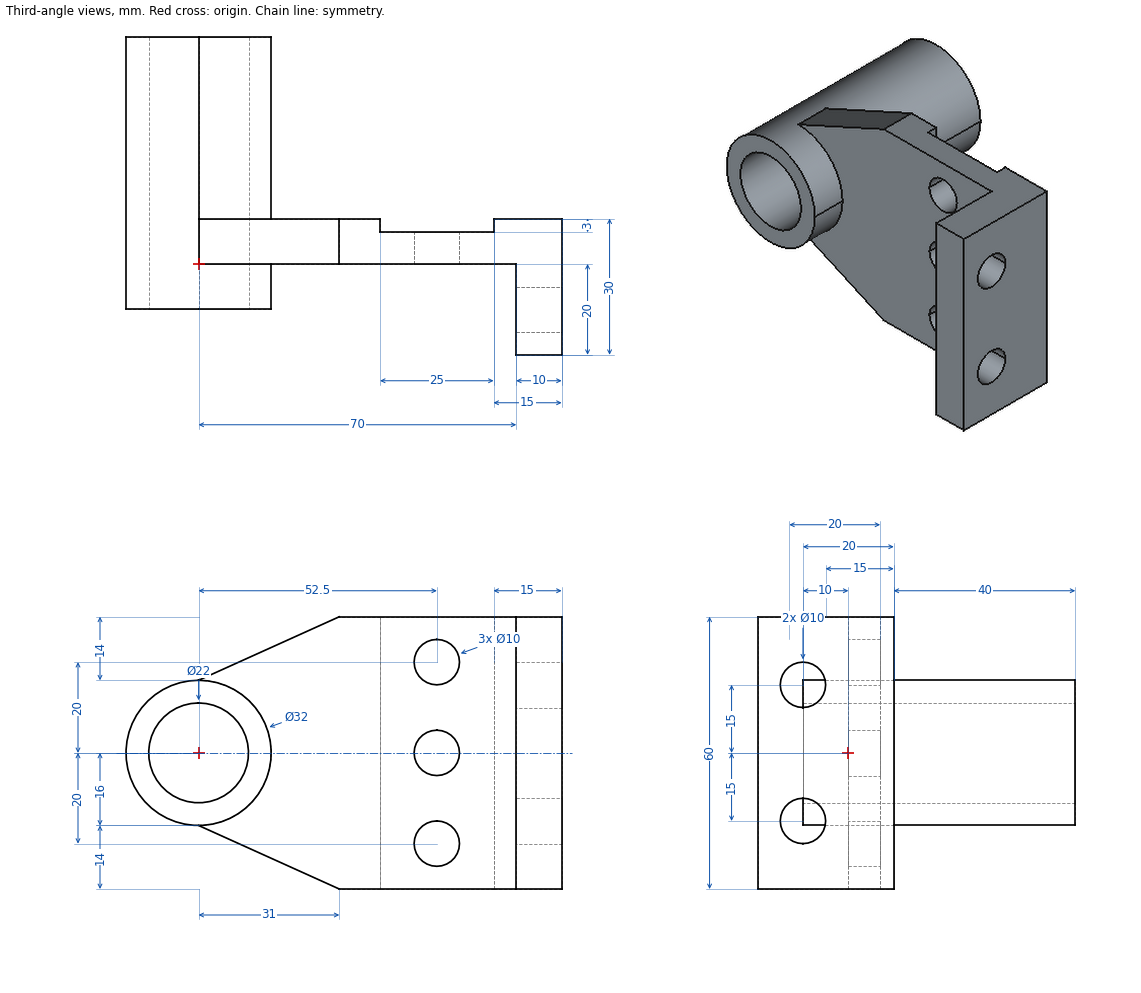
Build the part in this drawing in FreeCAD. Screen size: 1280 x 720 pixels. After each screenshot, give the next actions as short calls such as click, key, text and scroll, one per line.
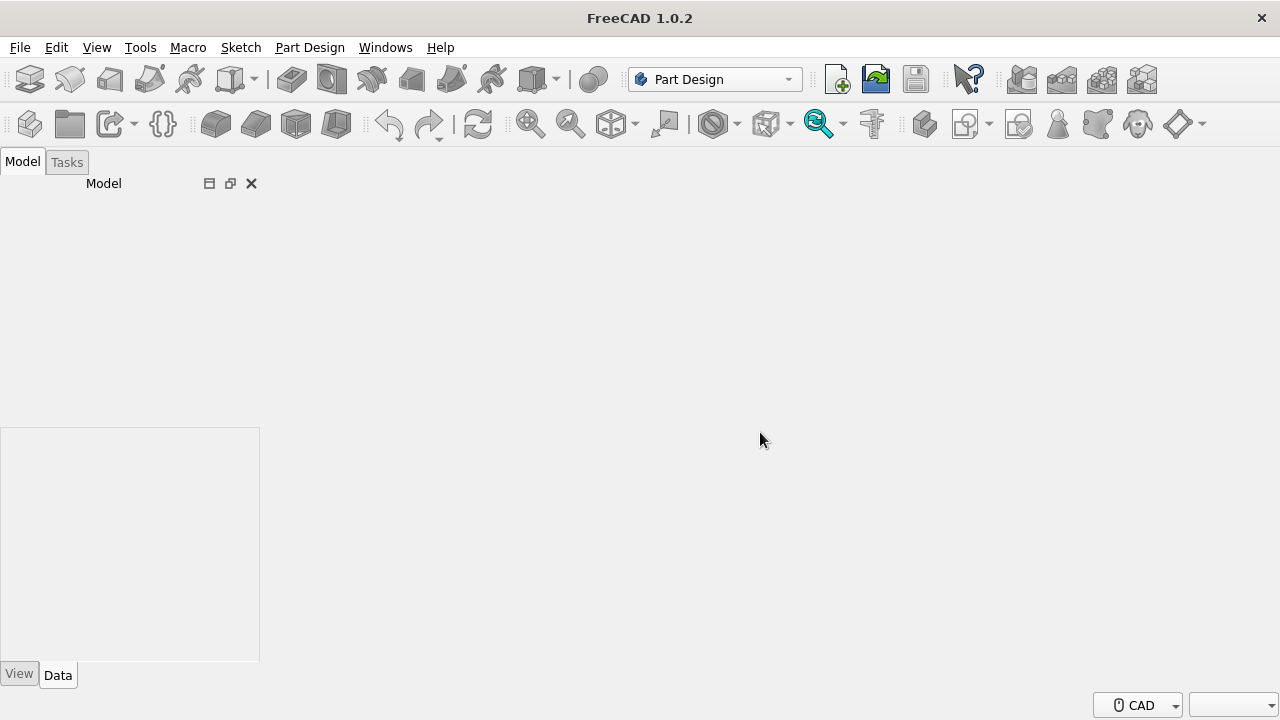
click(836, 80)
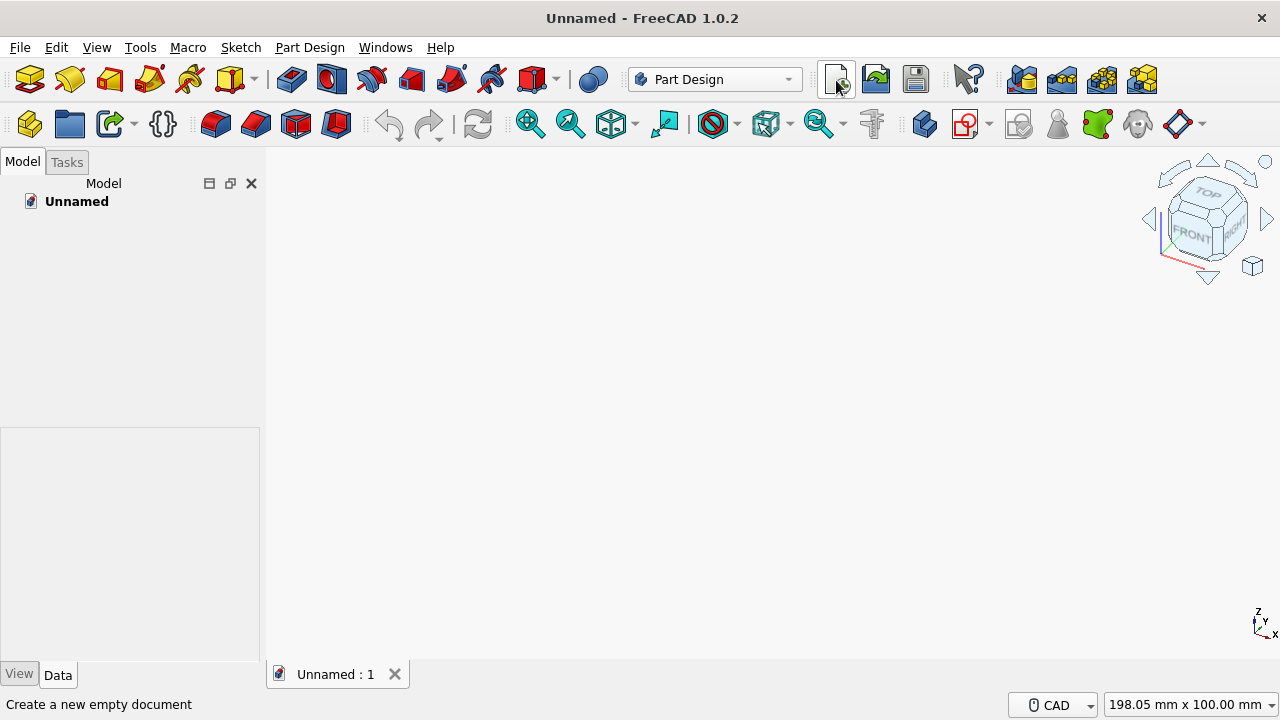
click(966, 124)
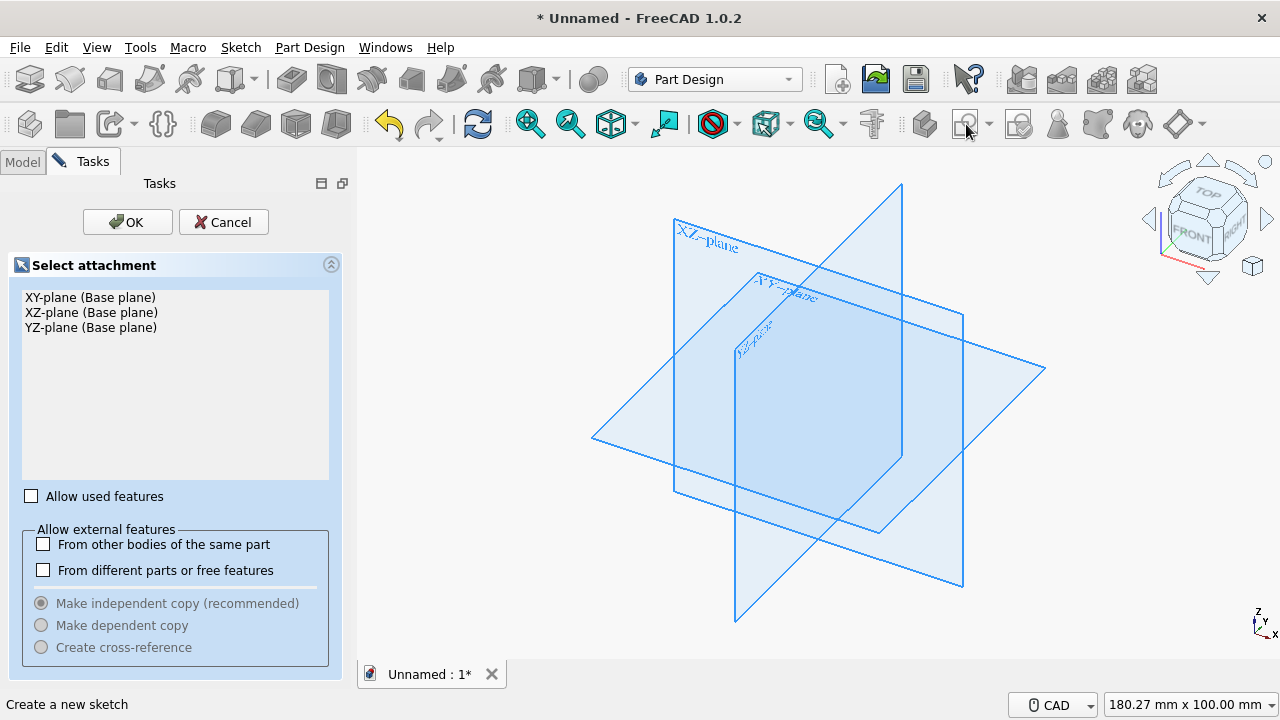
click(82, 298)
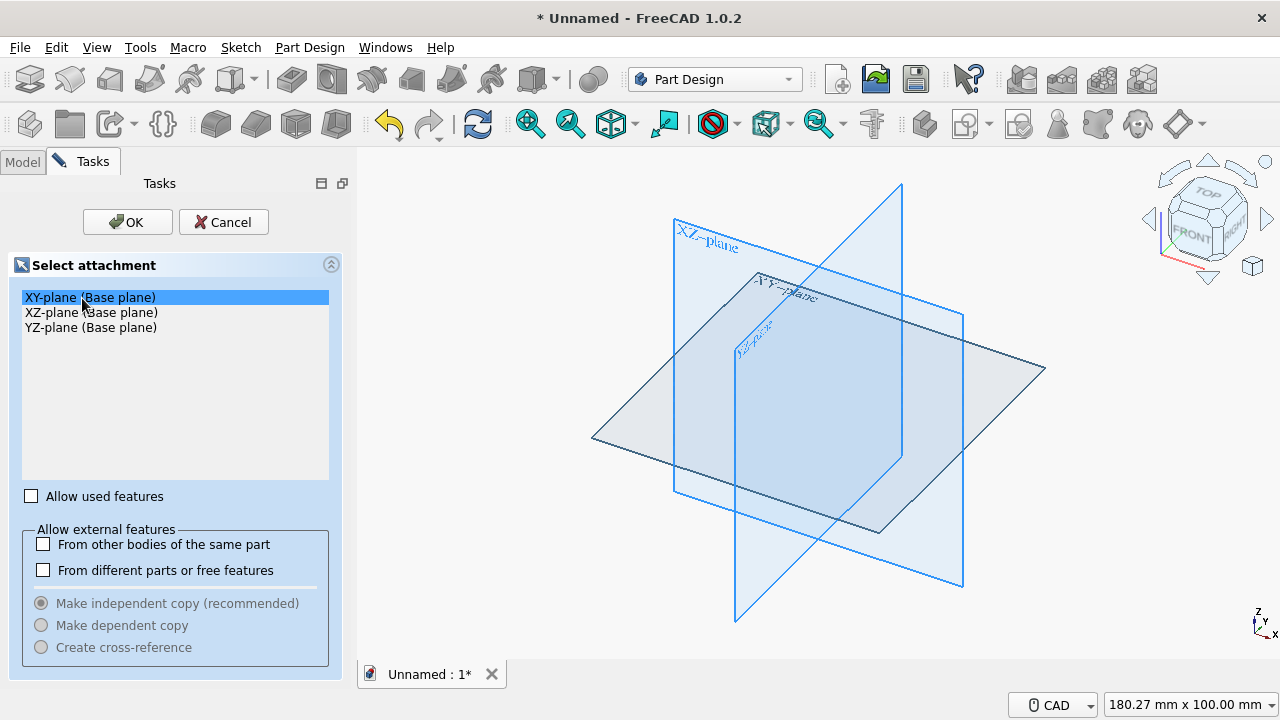
click(128, 222)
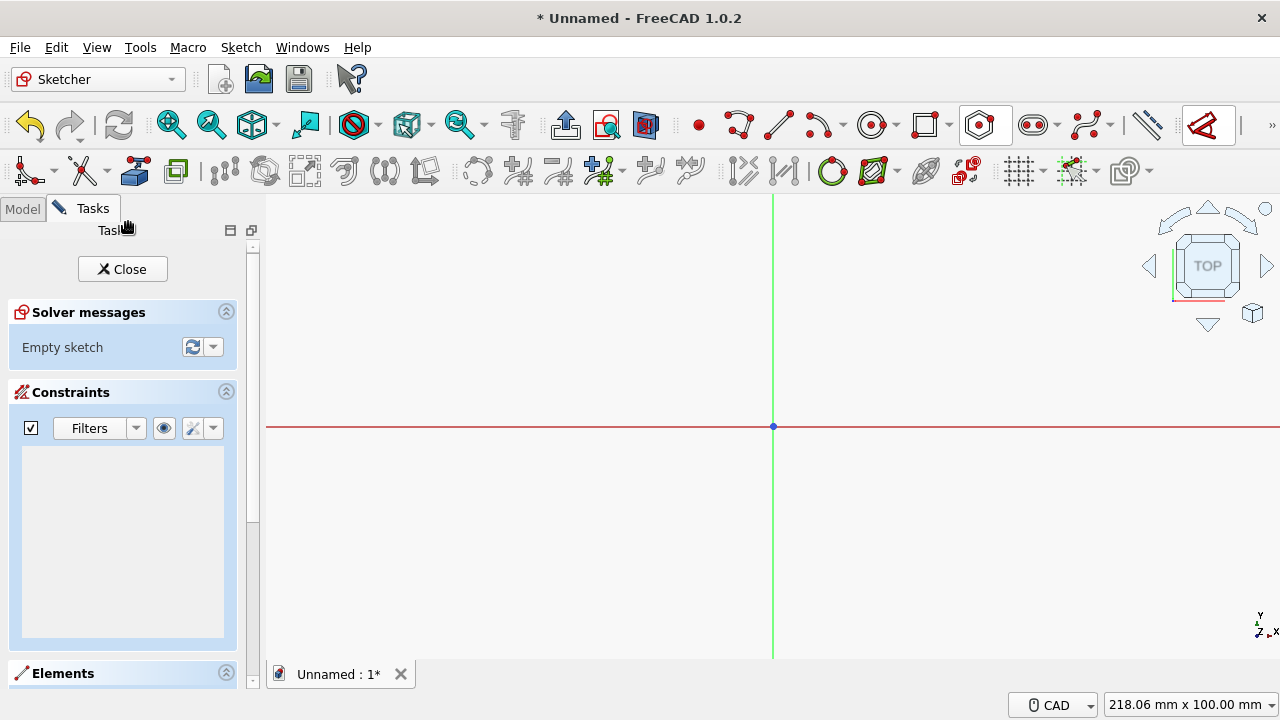
scroll(294, 321, down, 1)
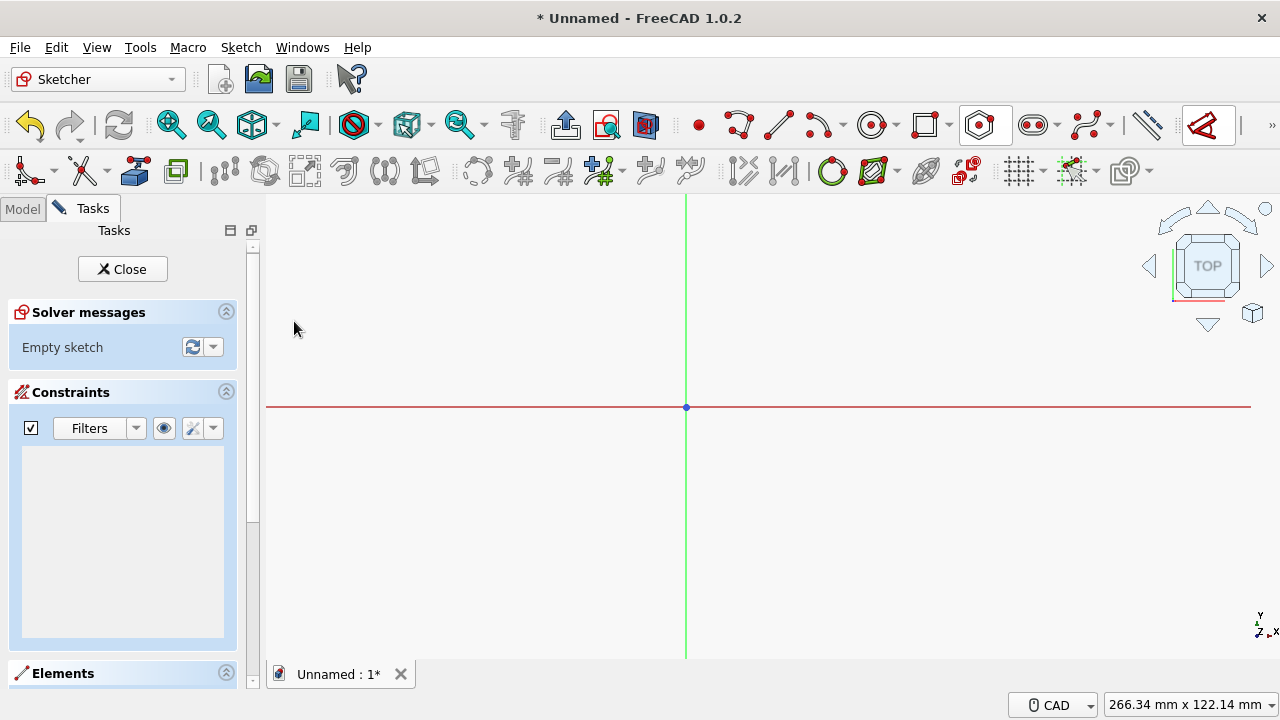
scroll(1001, 426, up, 3)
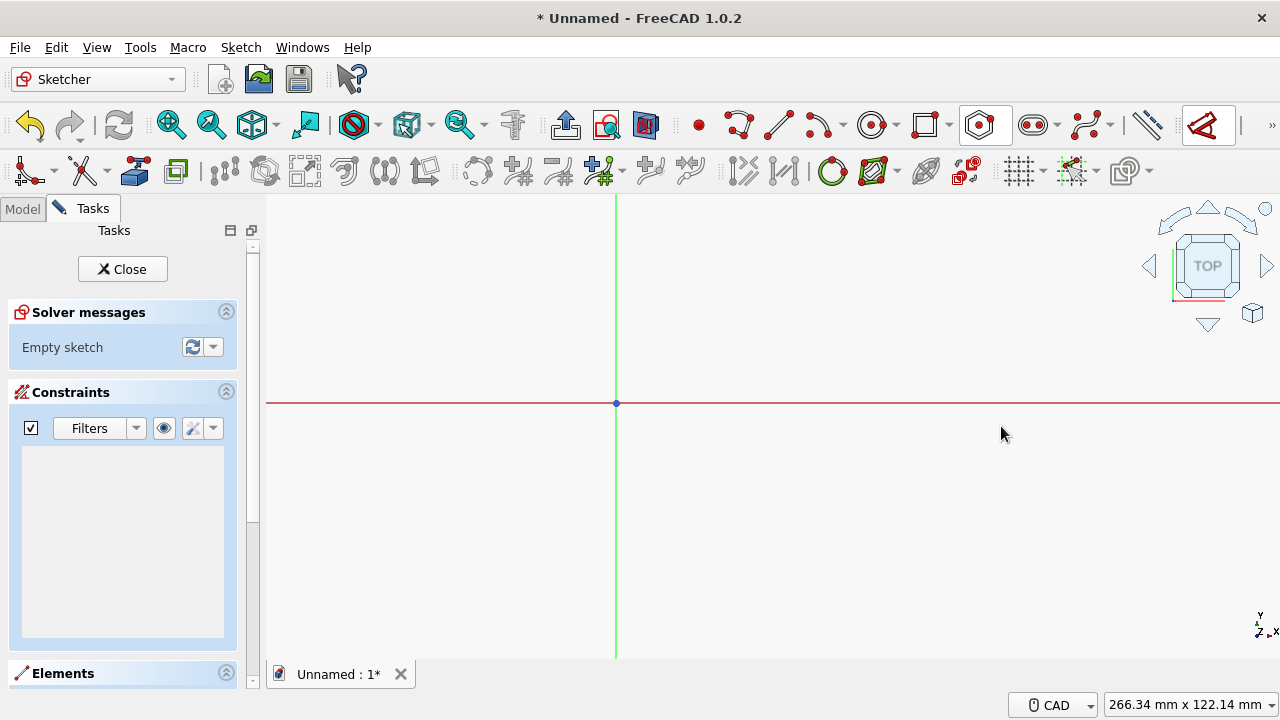
click(740, 126)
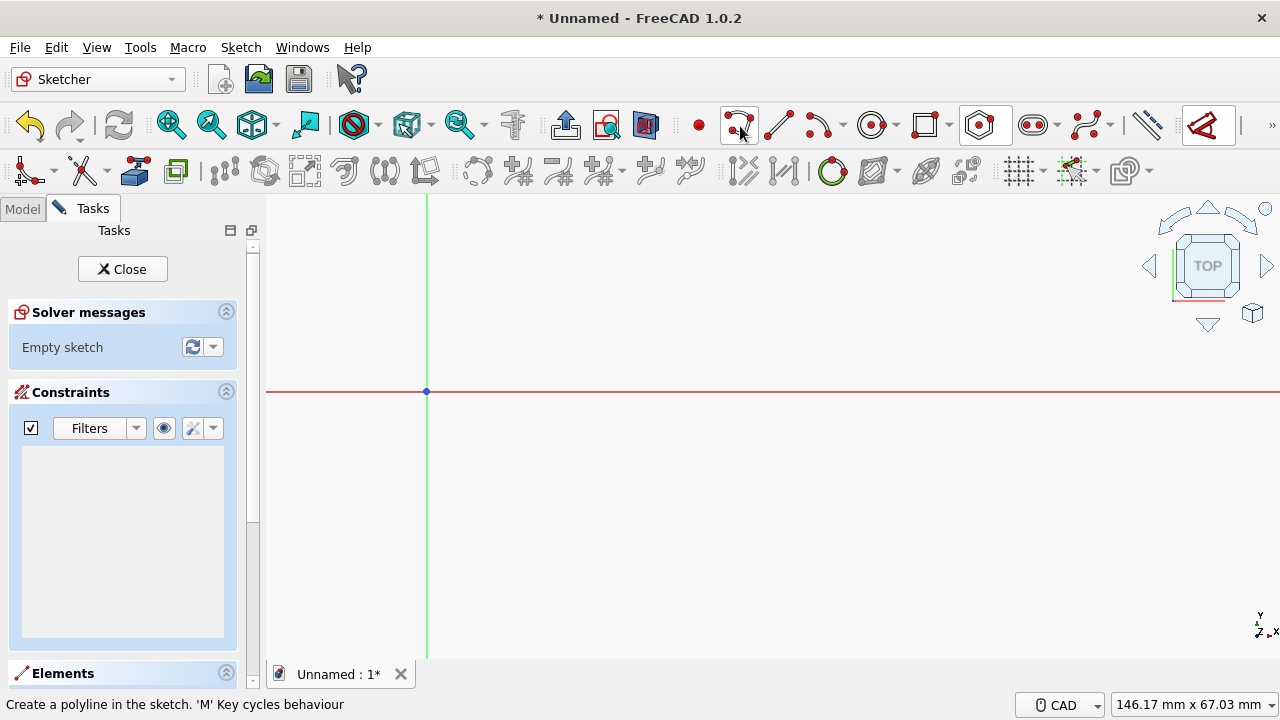
click(427, 392)
click(912, 401)
click(912, 530)
click(982, 530)
click(982, 322)
click(878, 322)
click(878, 343)
click(704, 343)
click(704, 322)
click(436, 322)
click(427, 392)
key(Escape)
key(Escape)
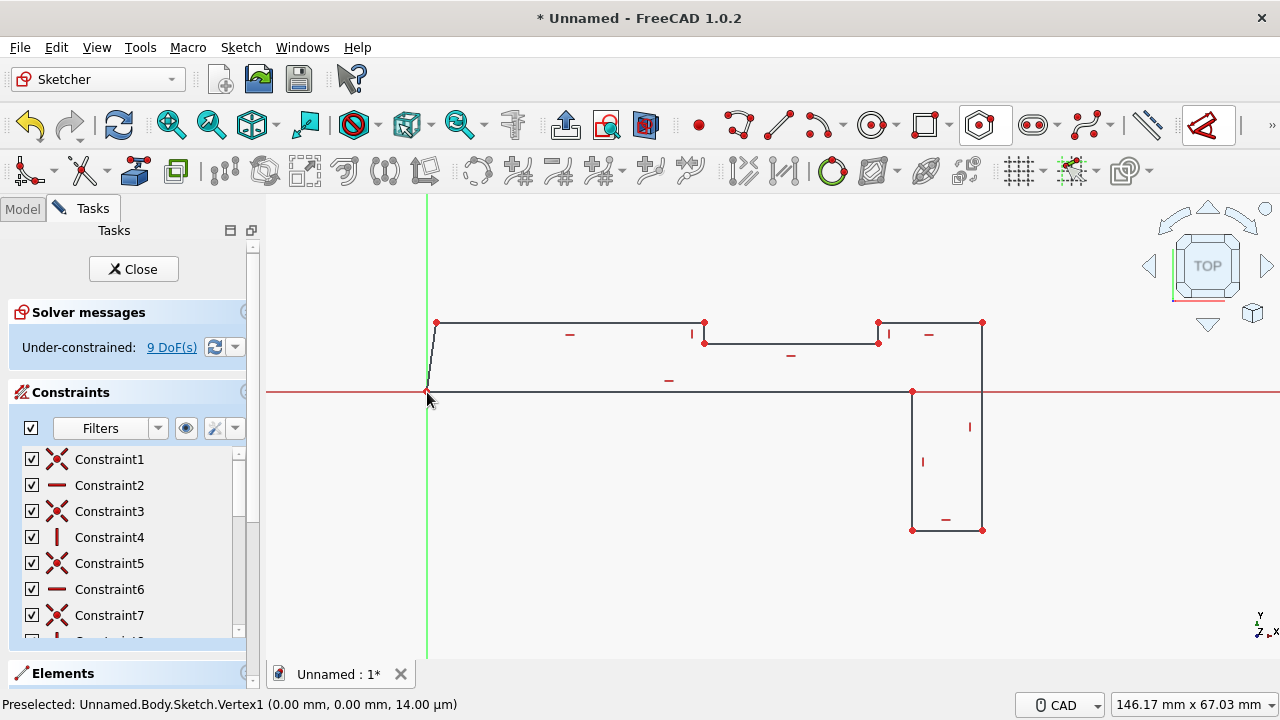
click(430, 371)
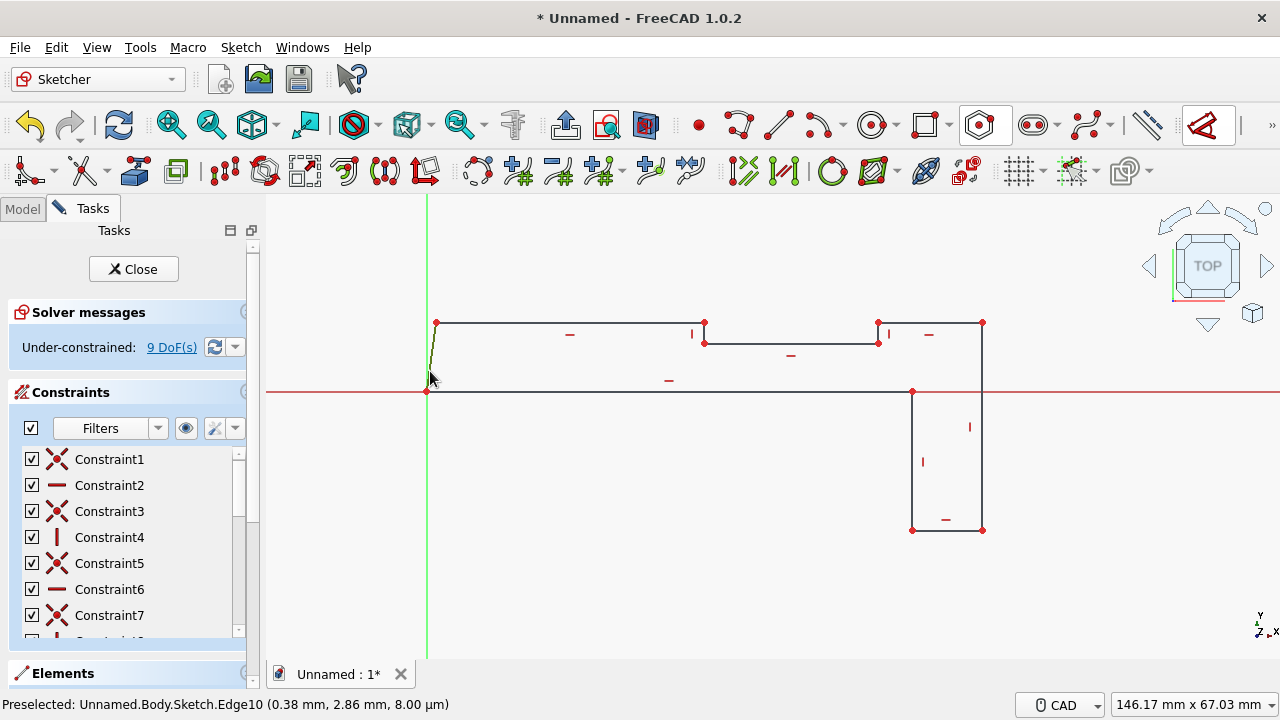
key(v)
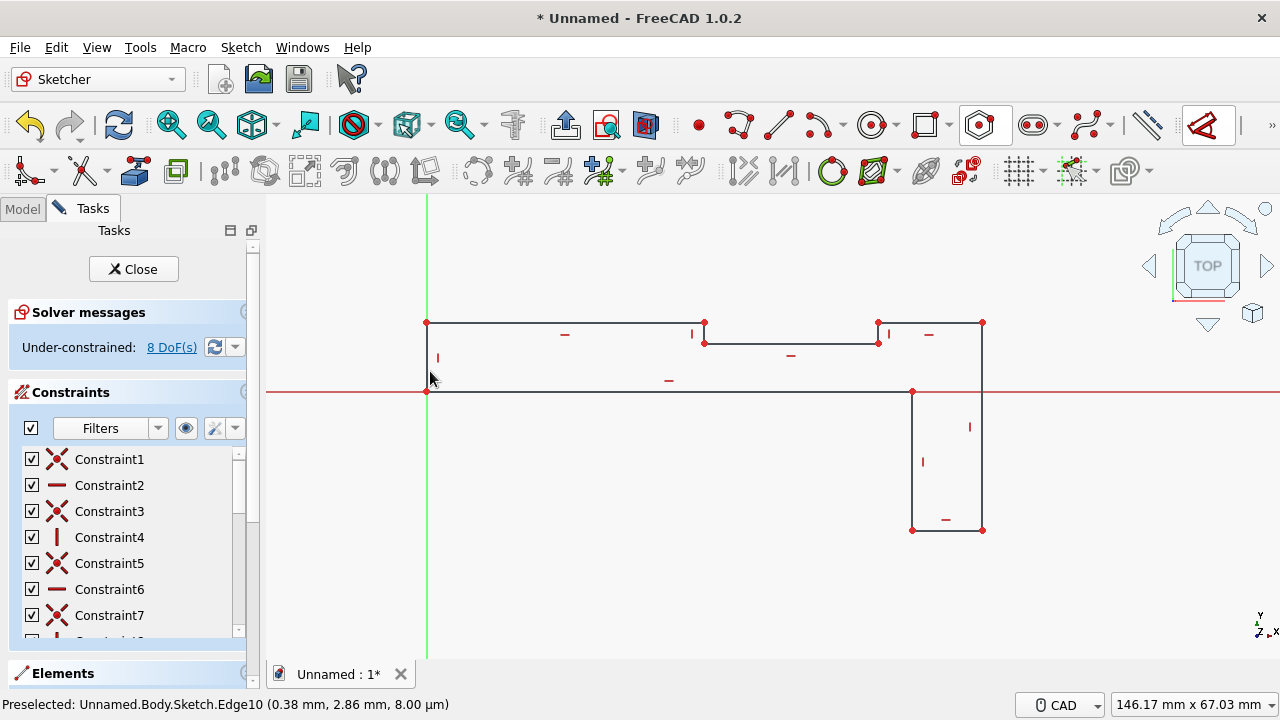
scroll(878, 333, up, 4)